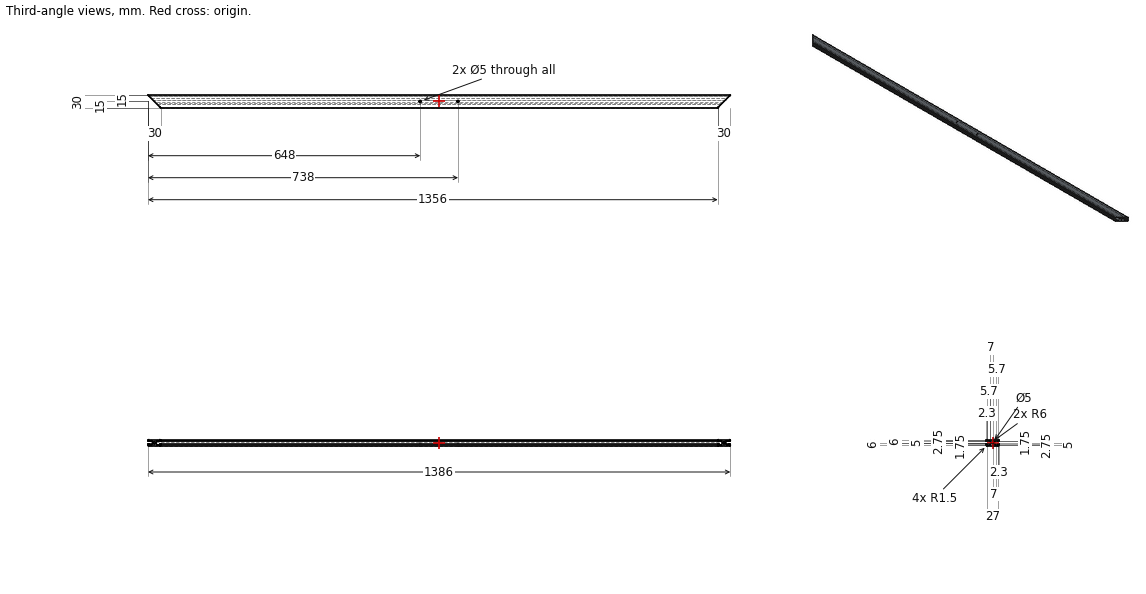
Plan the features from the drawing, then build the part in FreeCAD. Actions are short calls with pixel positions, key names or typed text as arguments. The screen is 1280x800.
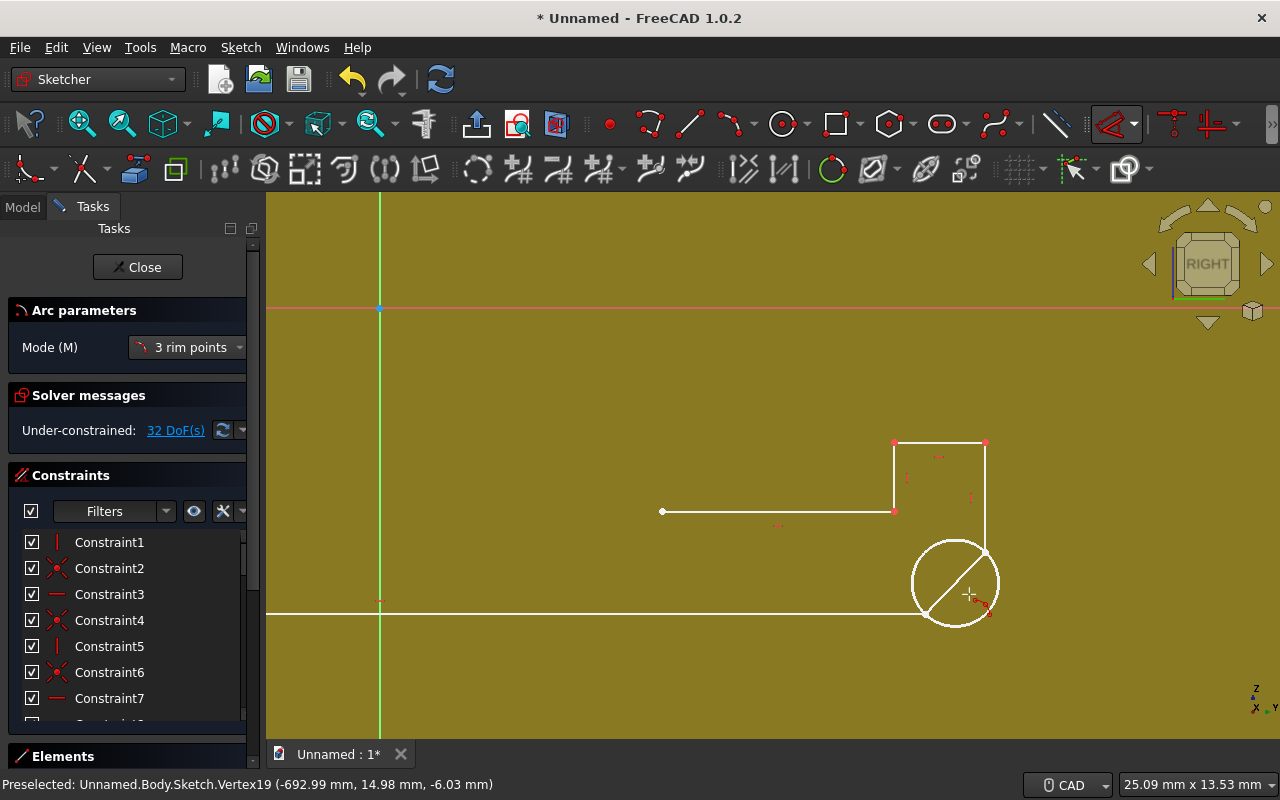
click(968, 594)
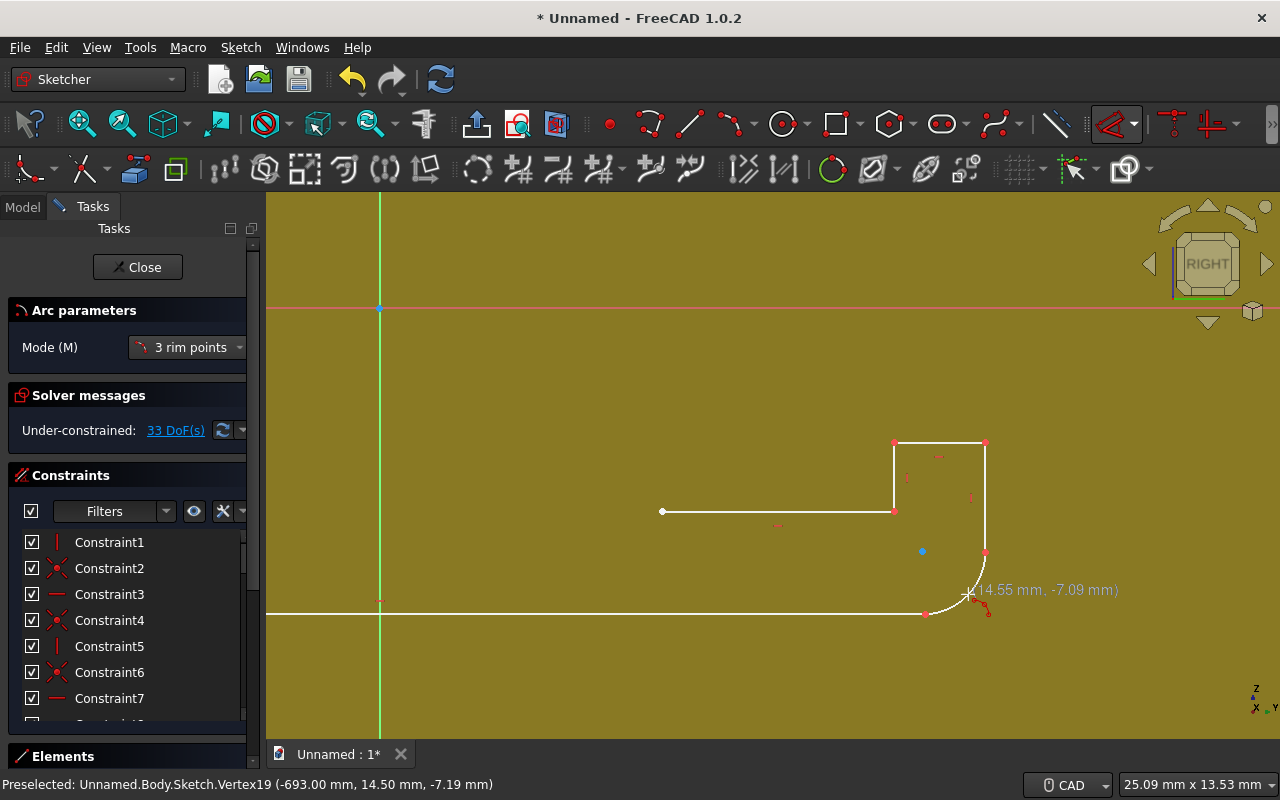
click(663, 512)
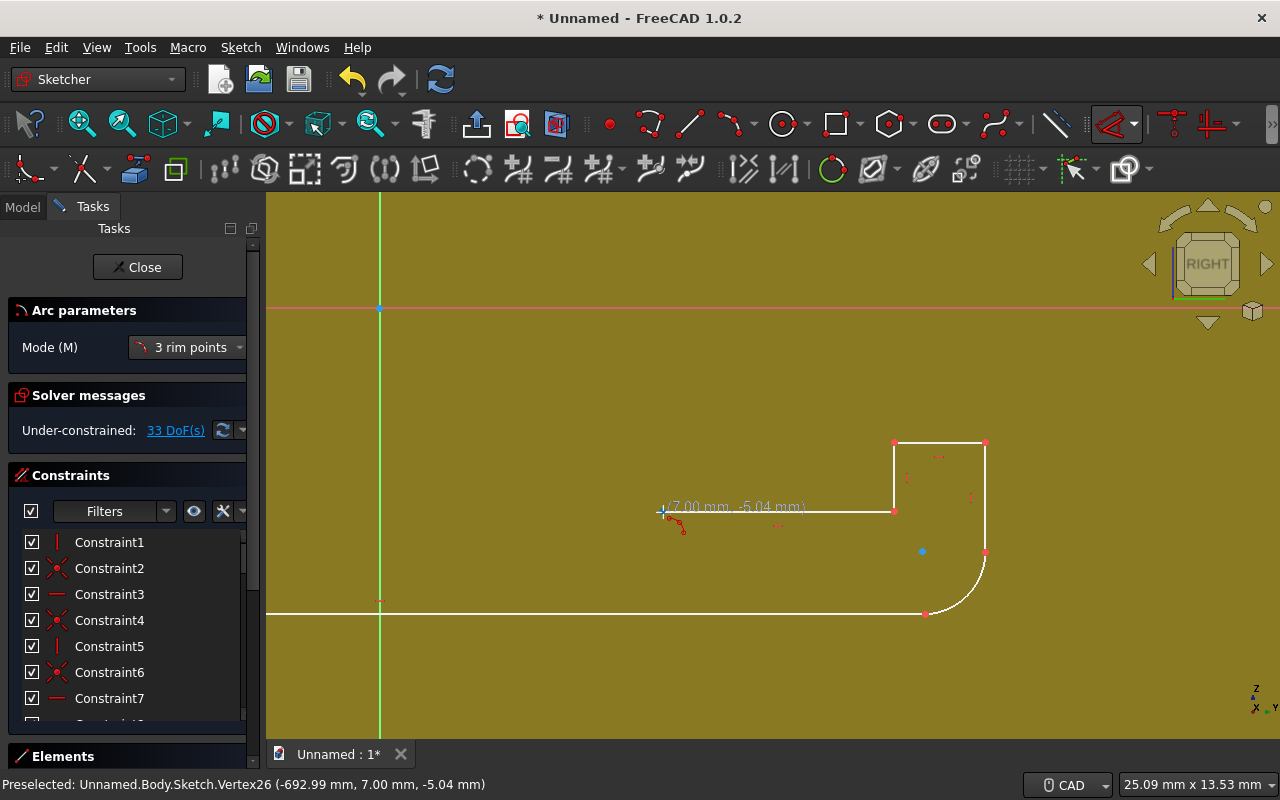
scroll(969, 594, down, 4)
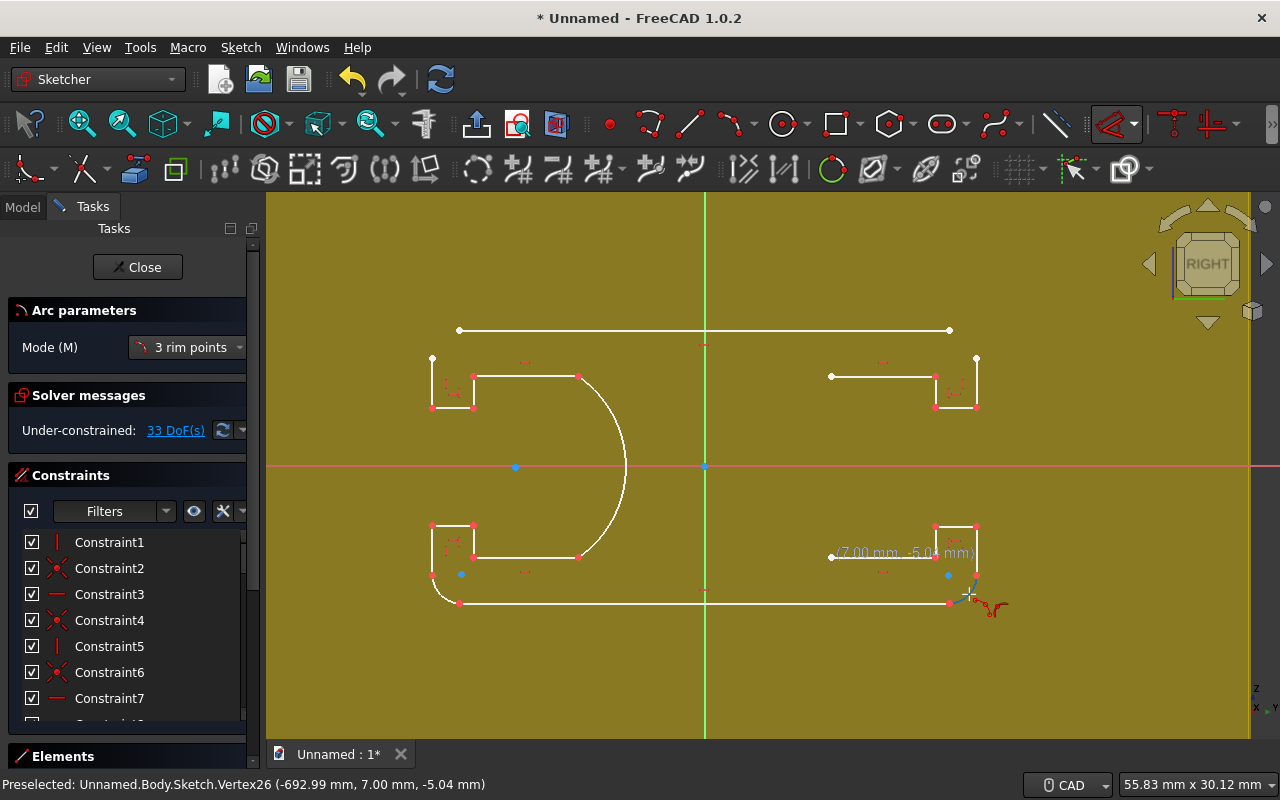
click(832, 377)
click(785, 445)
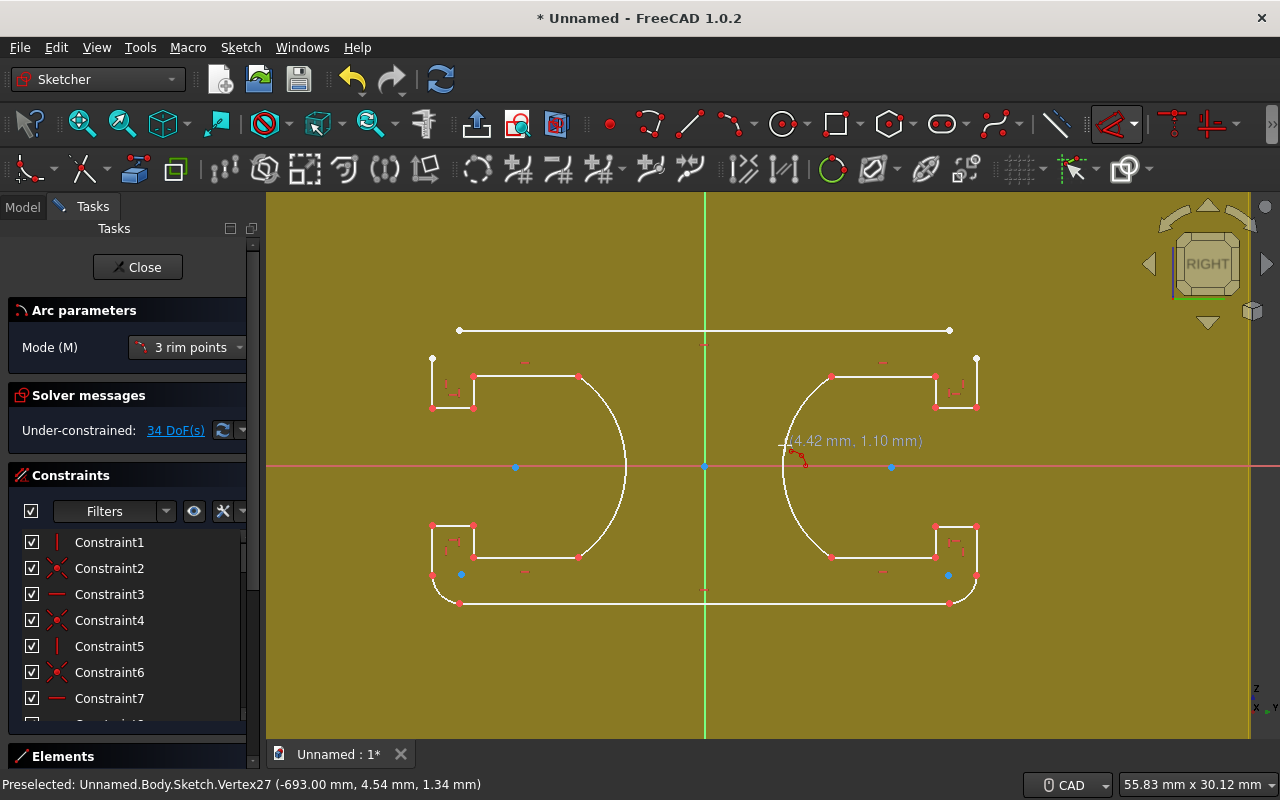
click(977, 359)
click(950, 331)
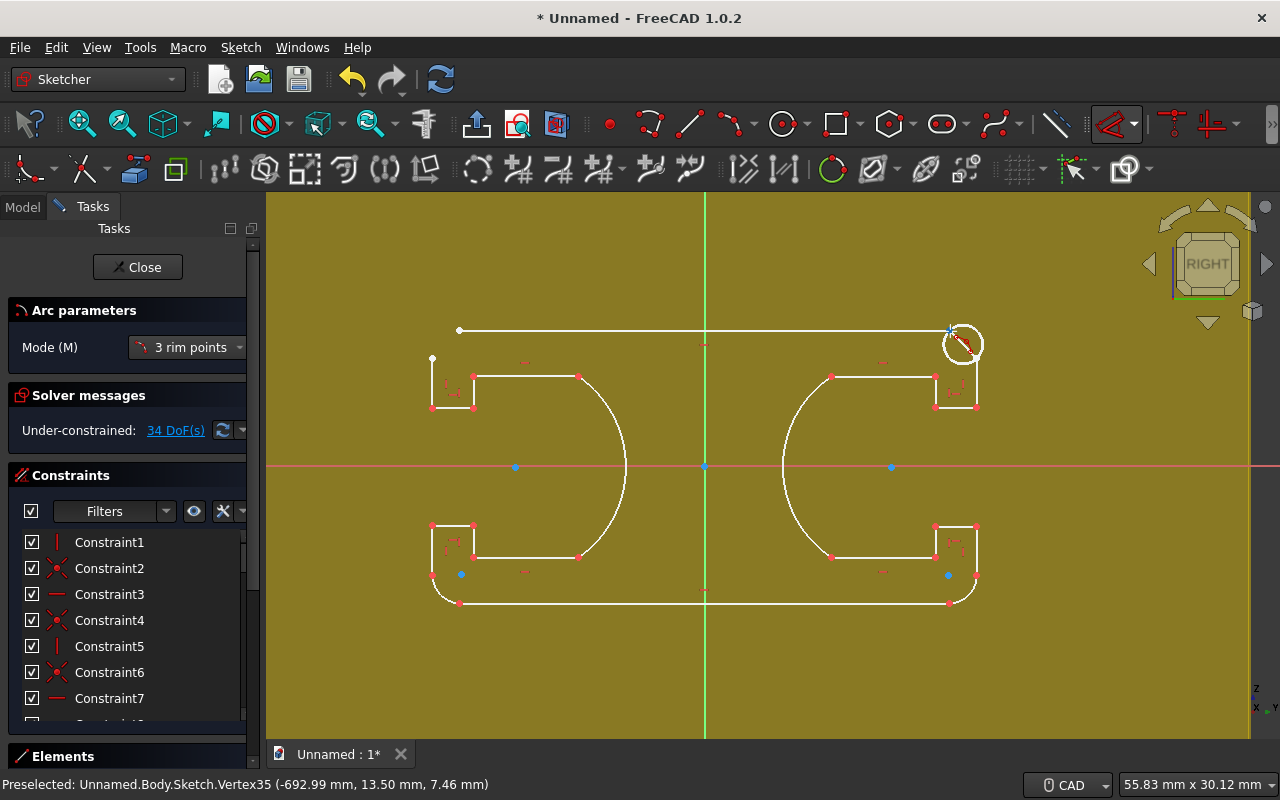
scroll(969, 338, up, 4)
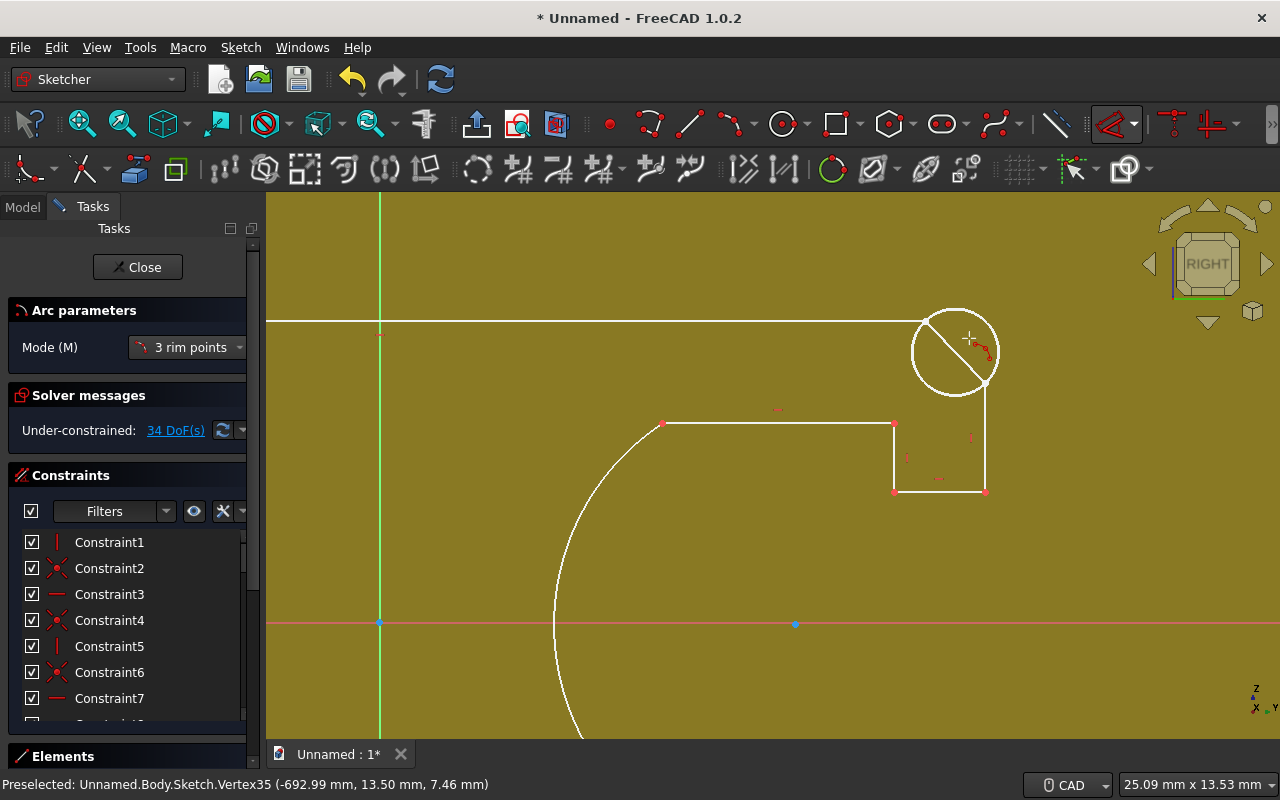
click(968, 337)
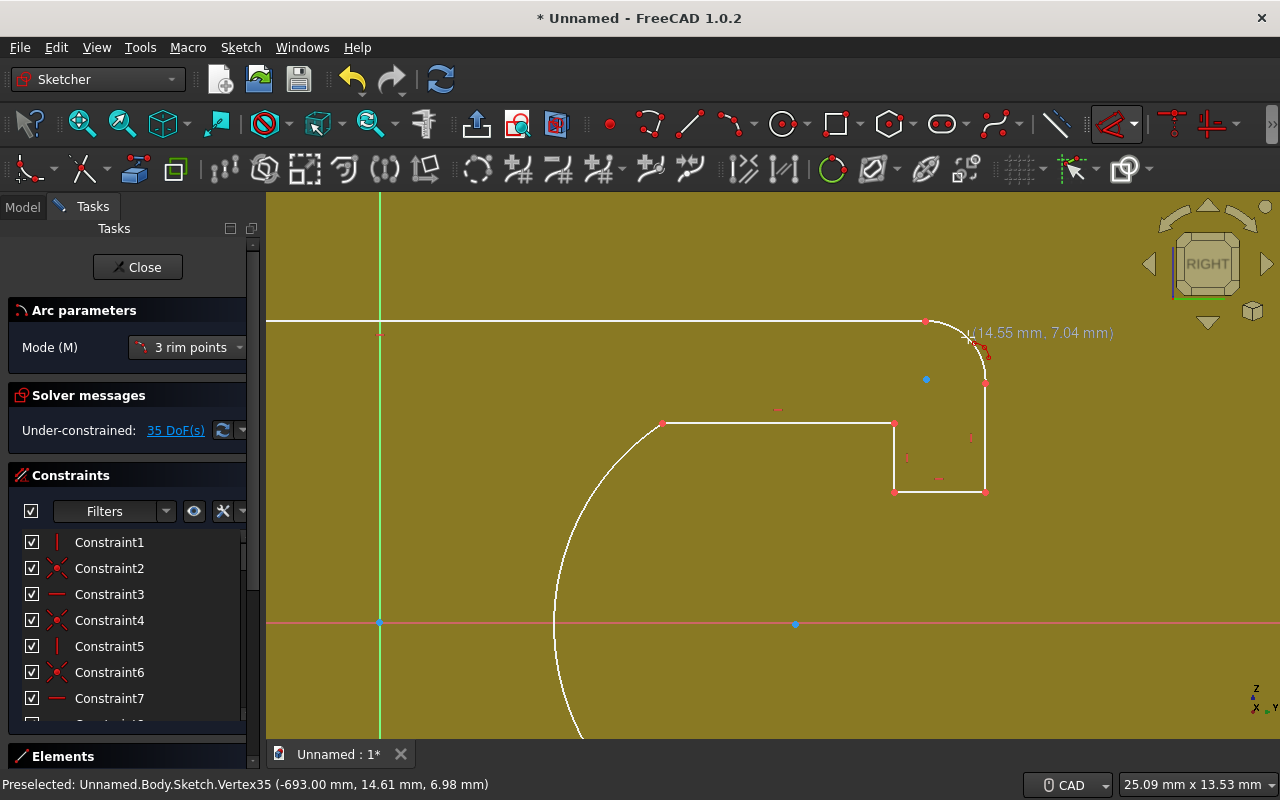
scroll(969, 337, down, 4)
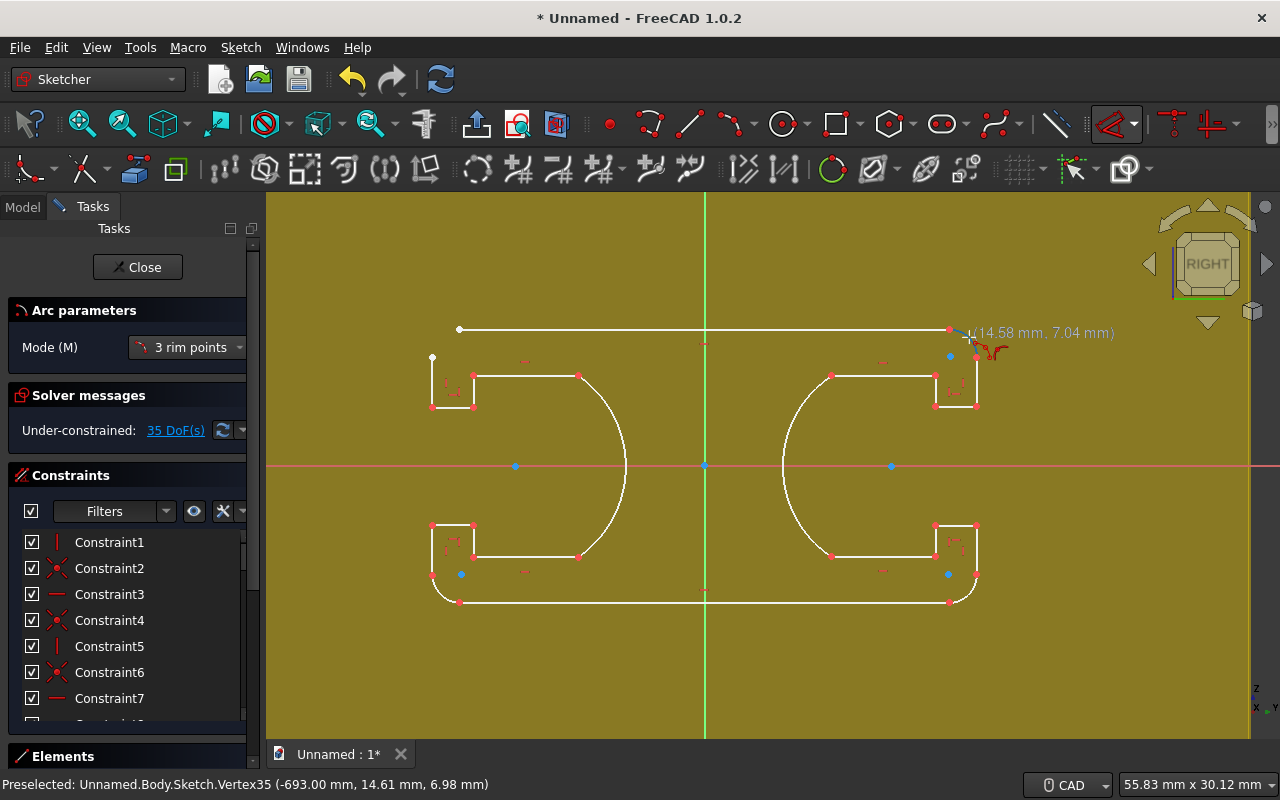
click(460, 330)
click(433, 358)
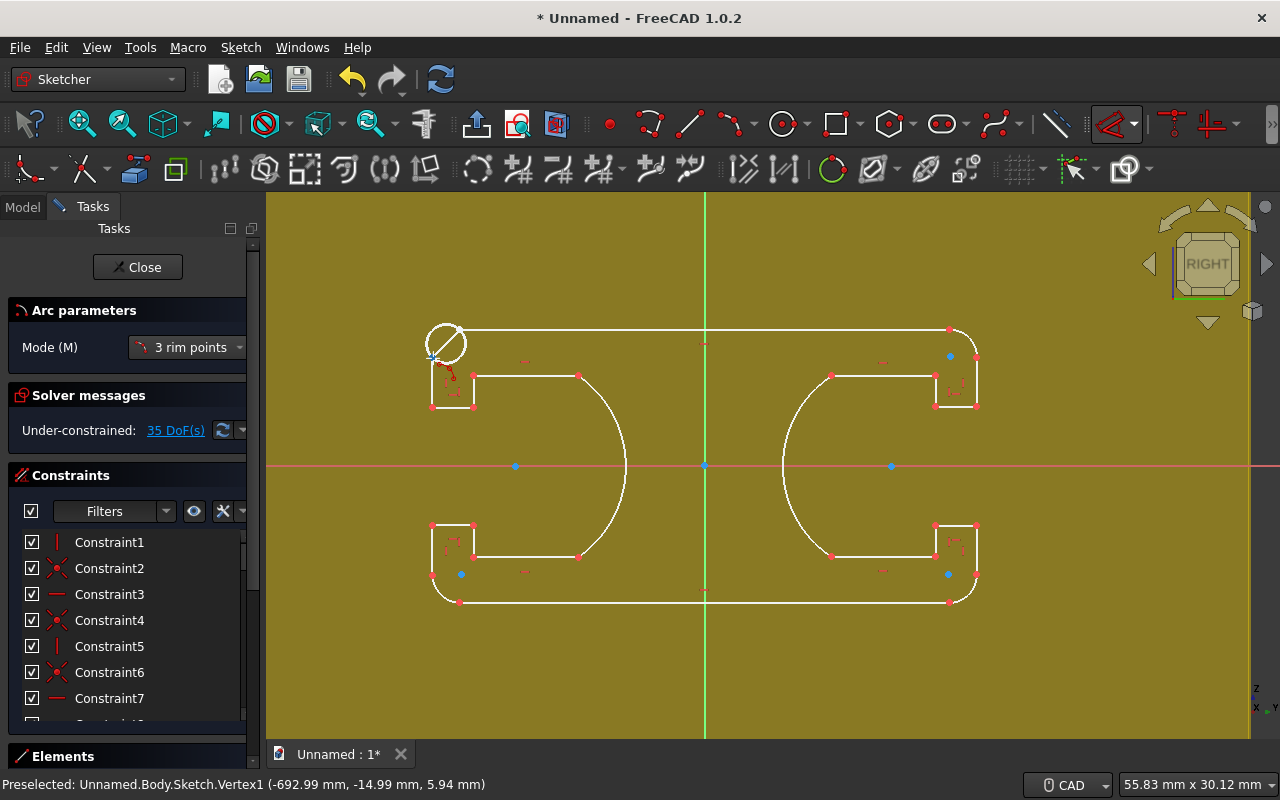
scroll(440, 337, up, 4)